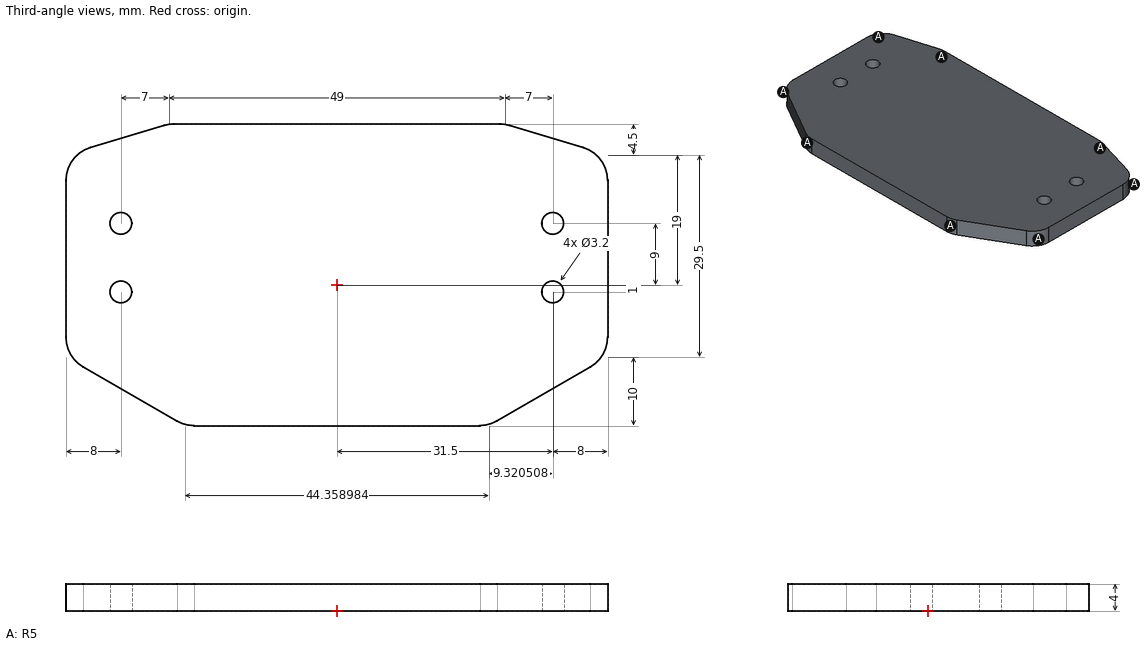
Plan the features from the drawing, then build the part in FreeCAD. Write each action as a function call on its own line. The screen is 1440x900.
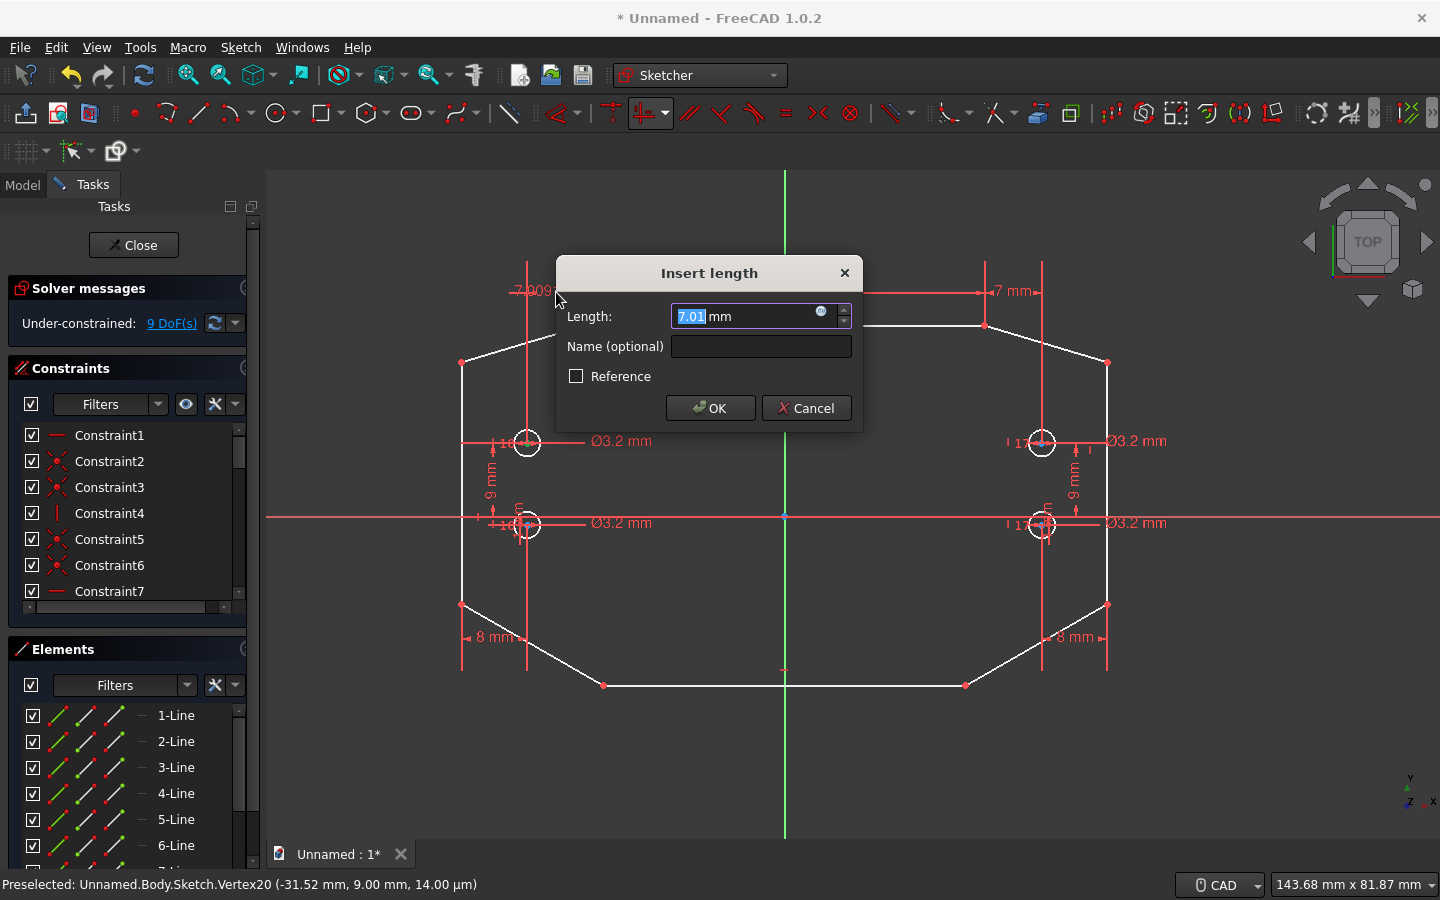
text(7)
key(Return)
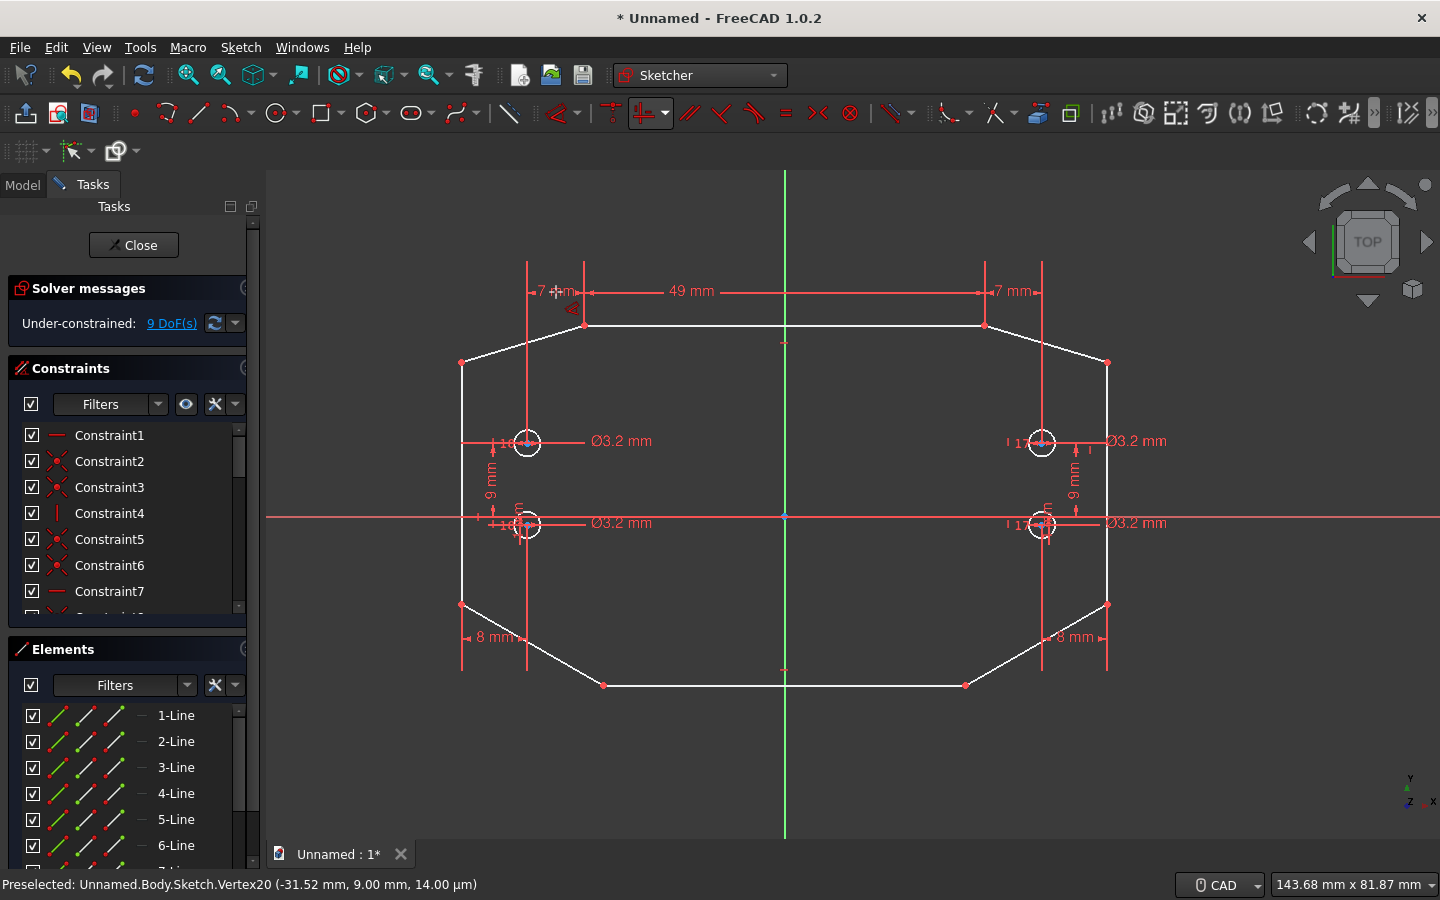
click(1107, 362)
click(1141, 440)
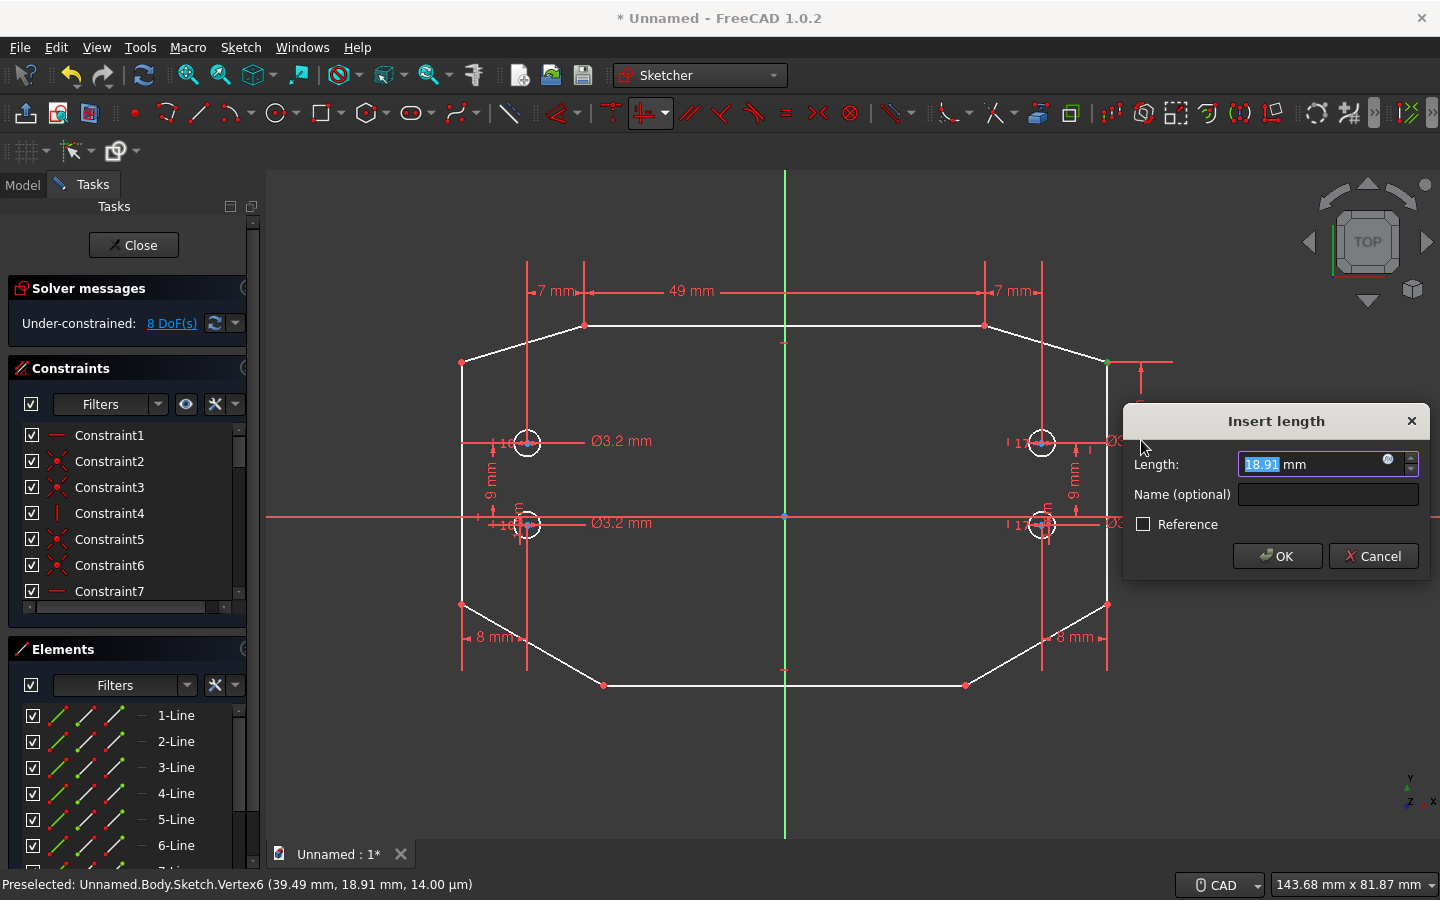
text(19)
key(Return)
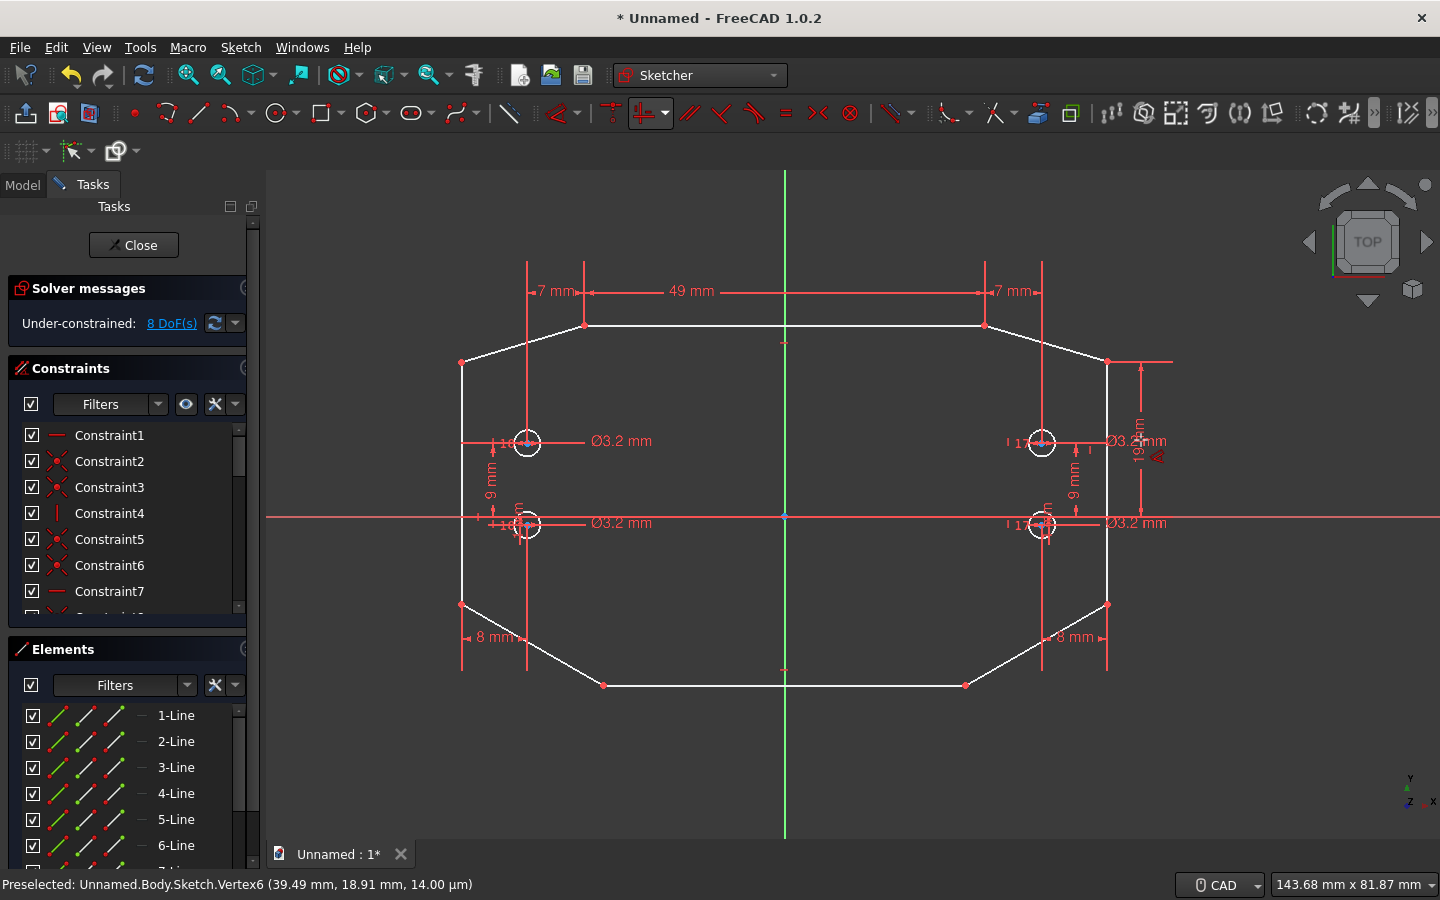
click(462, 362)
click(428, 440)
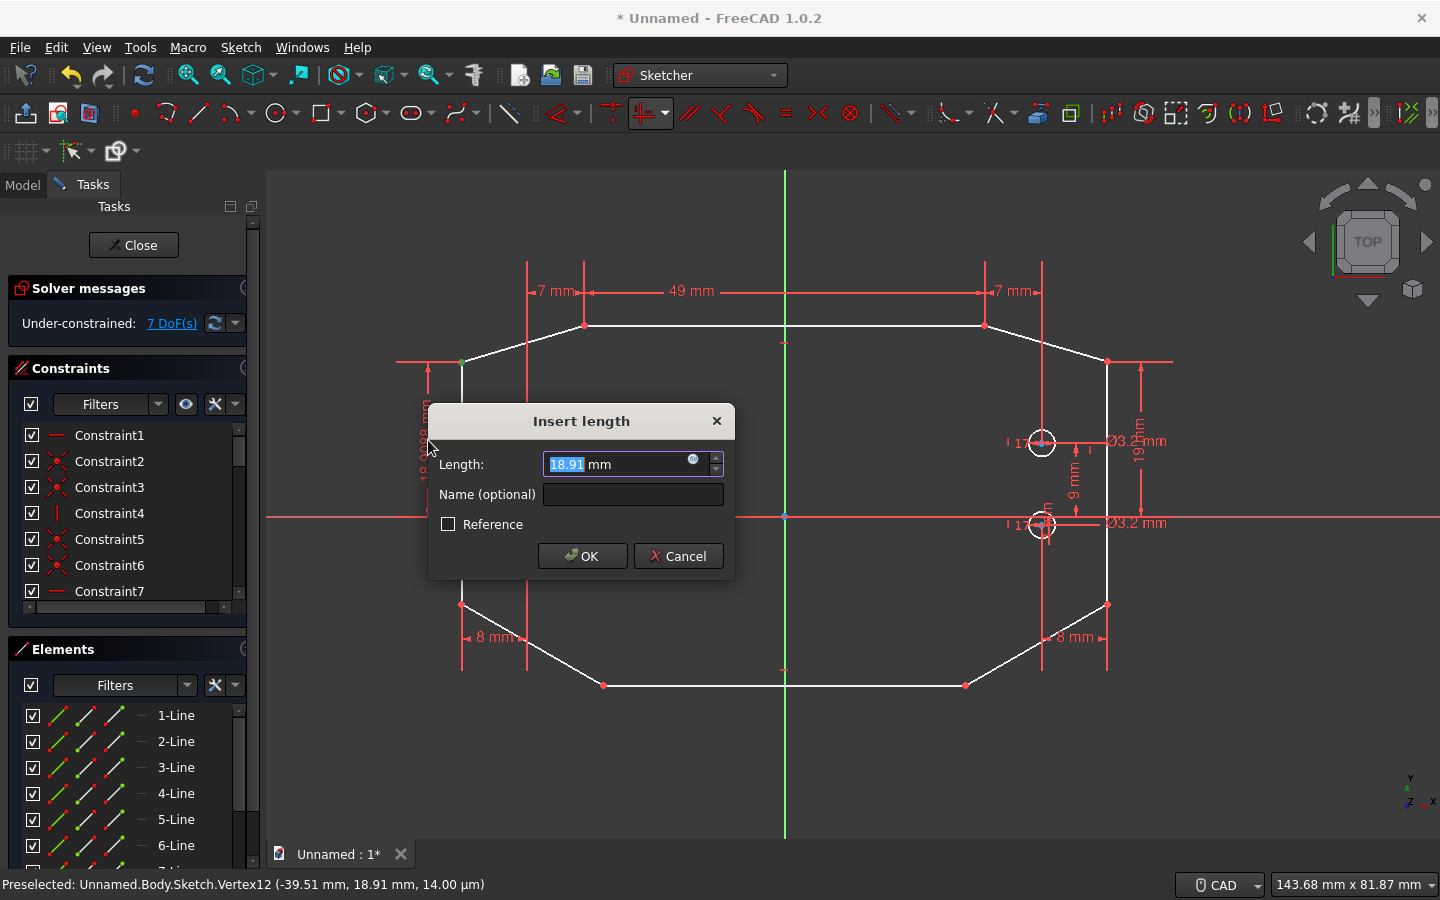
text(19)
key(Return)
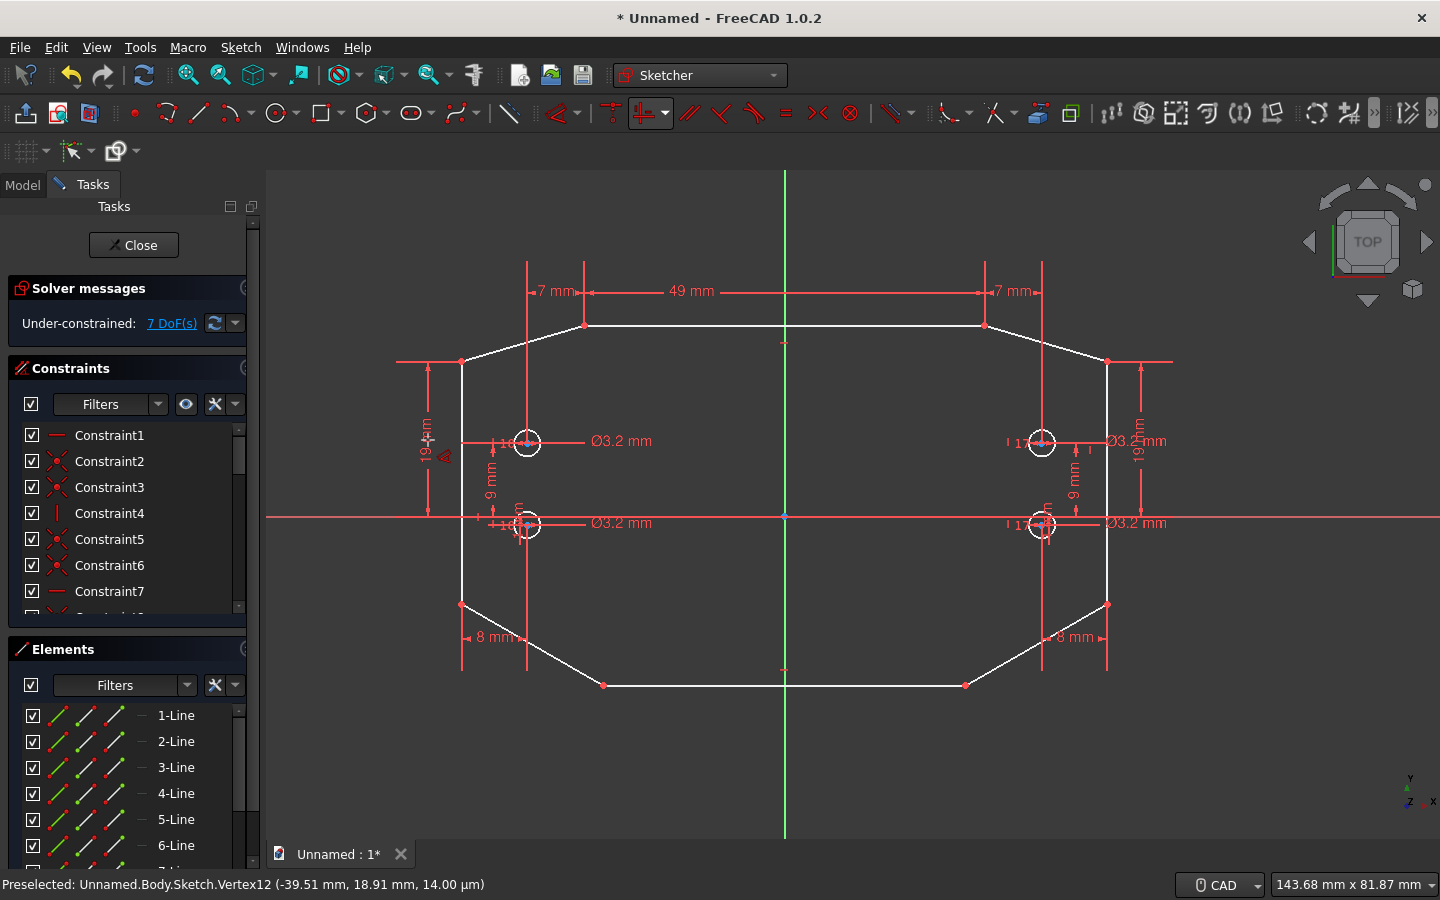
click(1008, 661)
click(1141, 664)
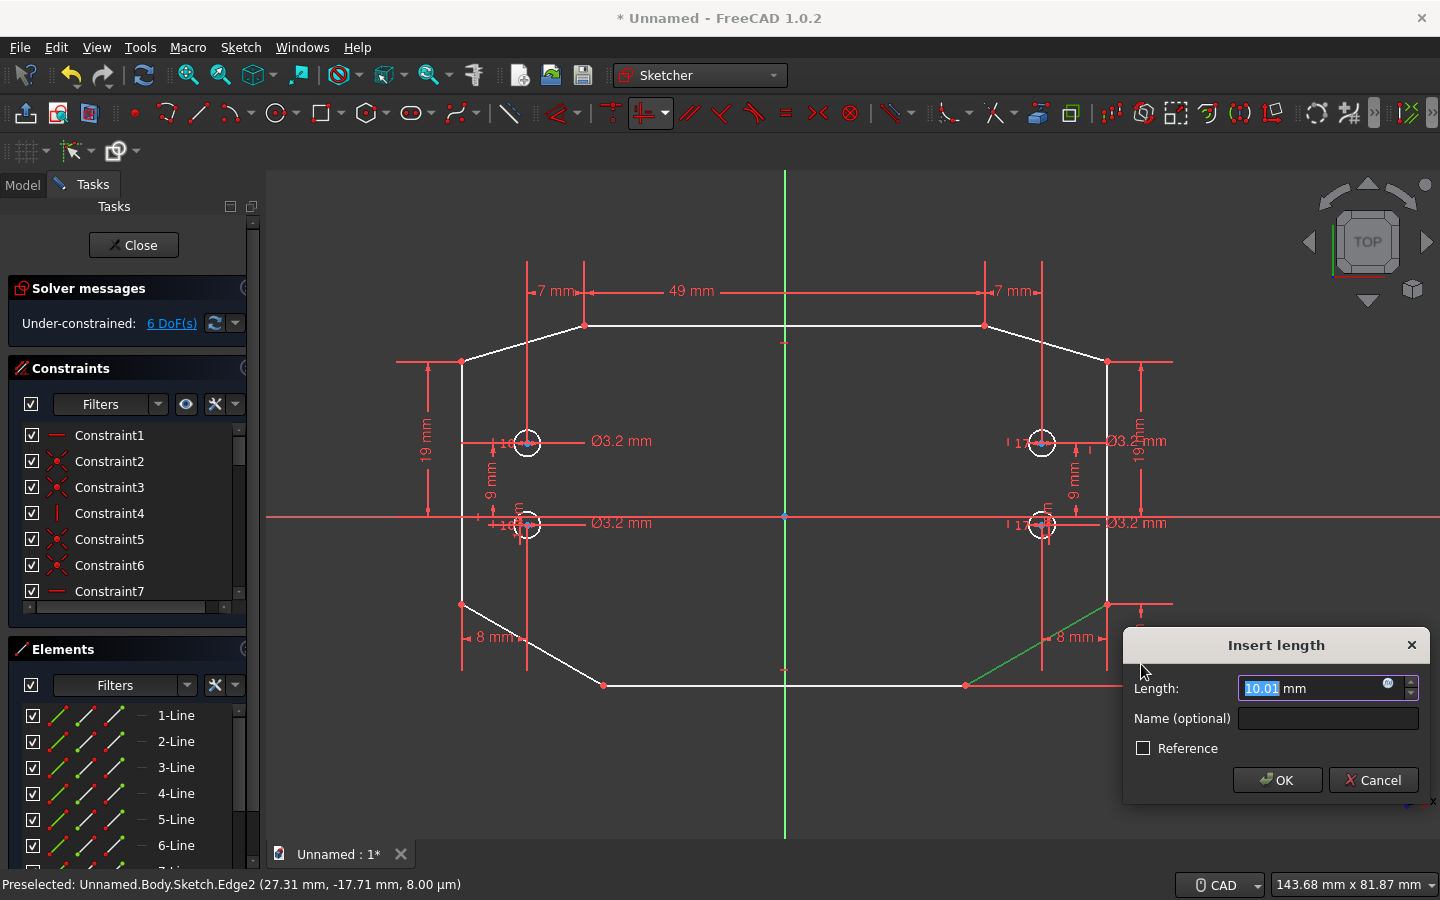
text(10)
key(Return)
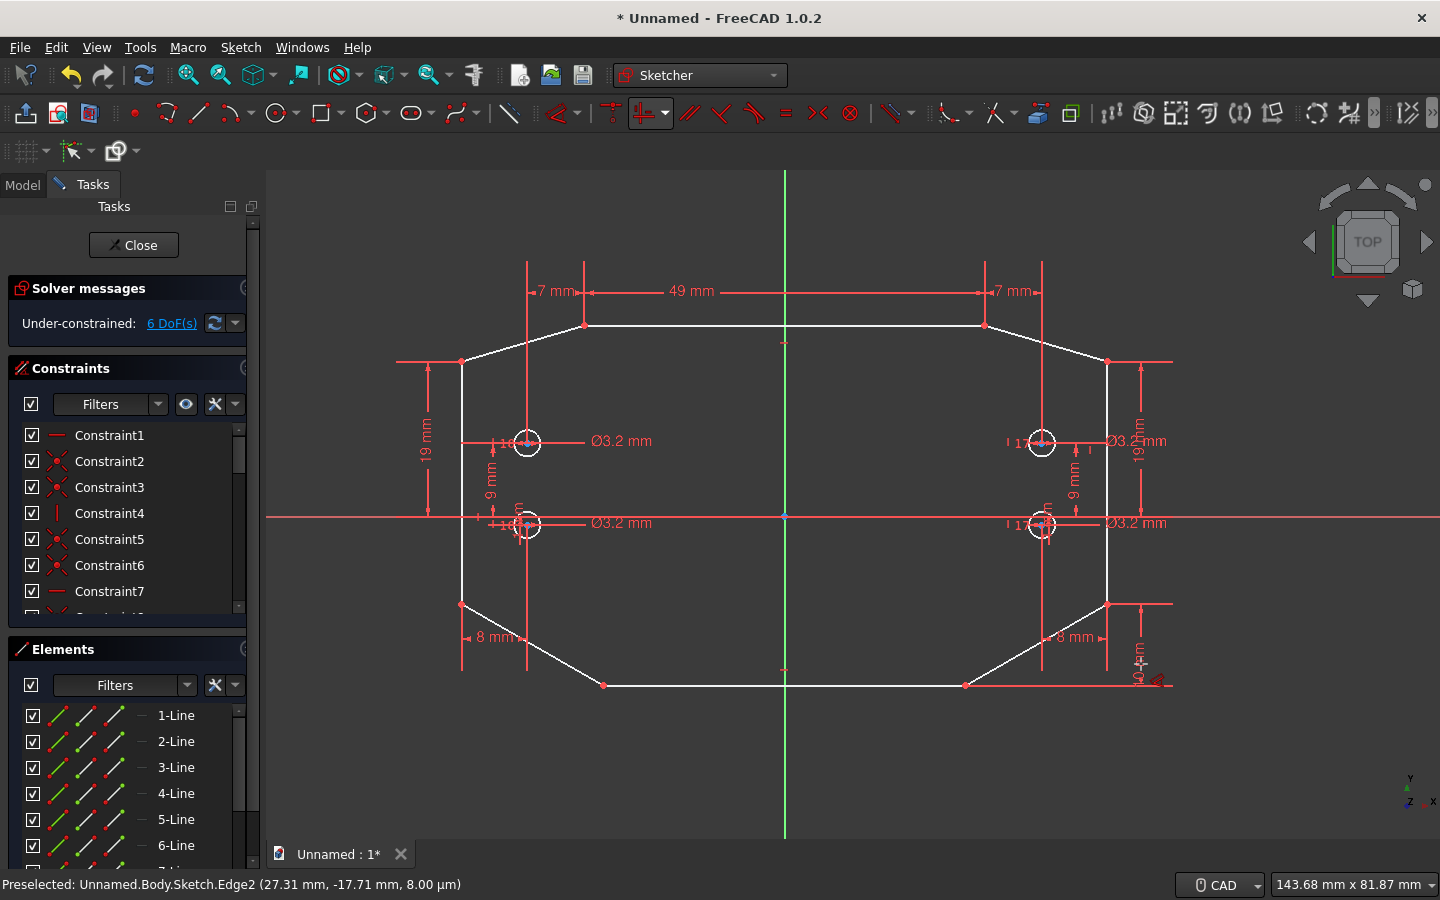
click(504, 629)
click(428, 664)